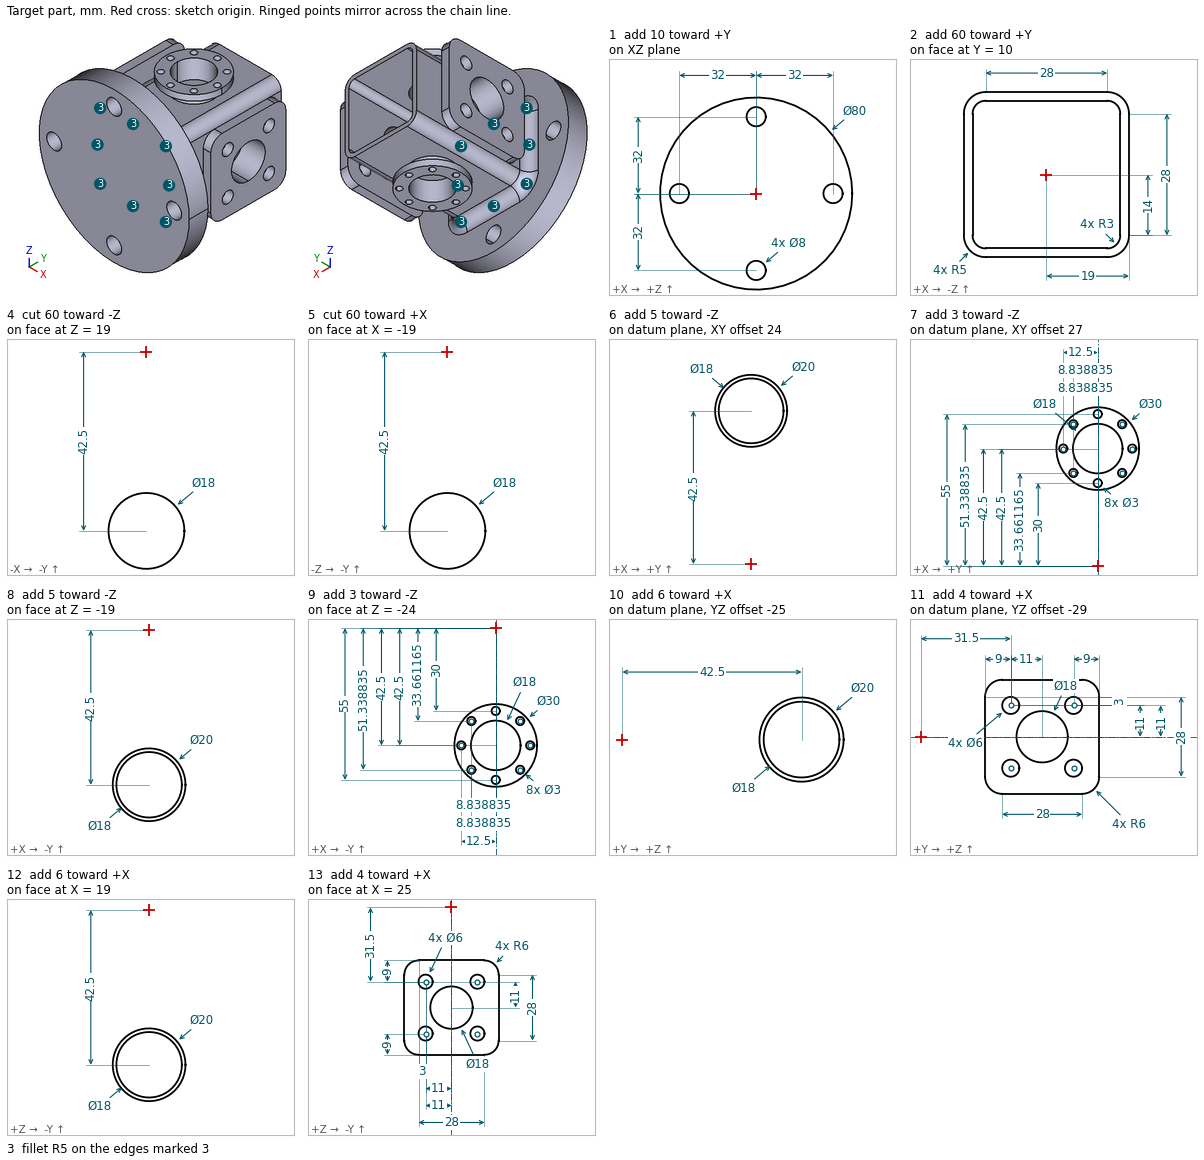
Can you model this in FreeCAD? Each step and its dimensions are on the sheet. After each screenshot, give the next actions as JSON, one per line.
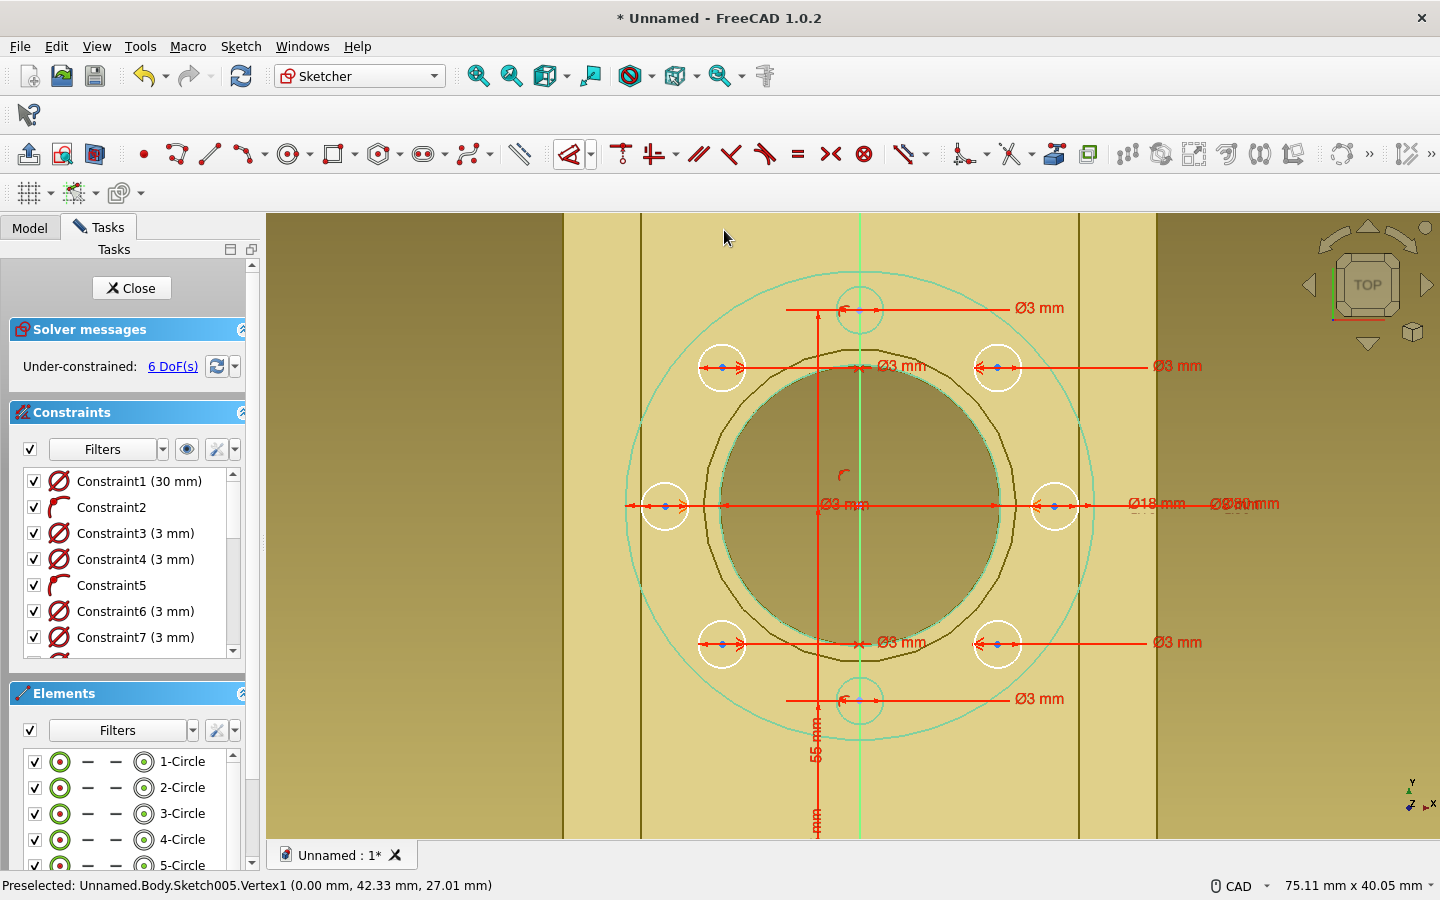
{"action": "left_click", "coordinate": [665, 506]}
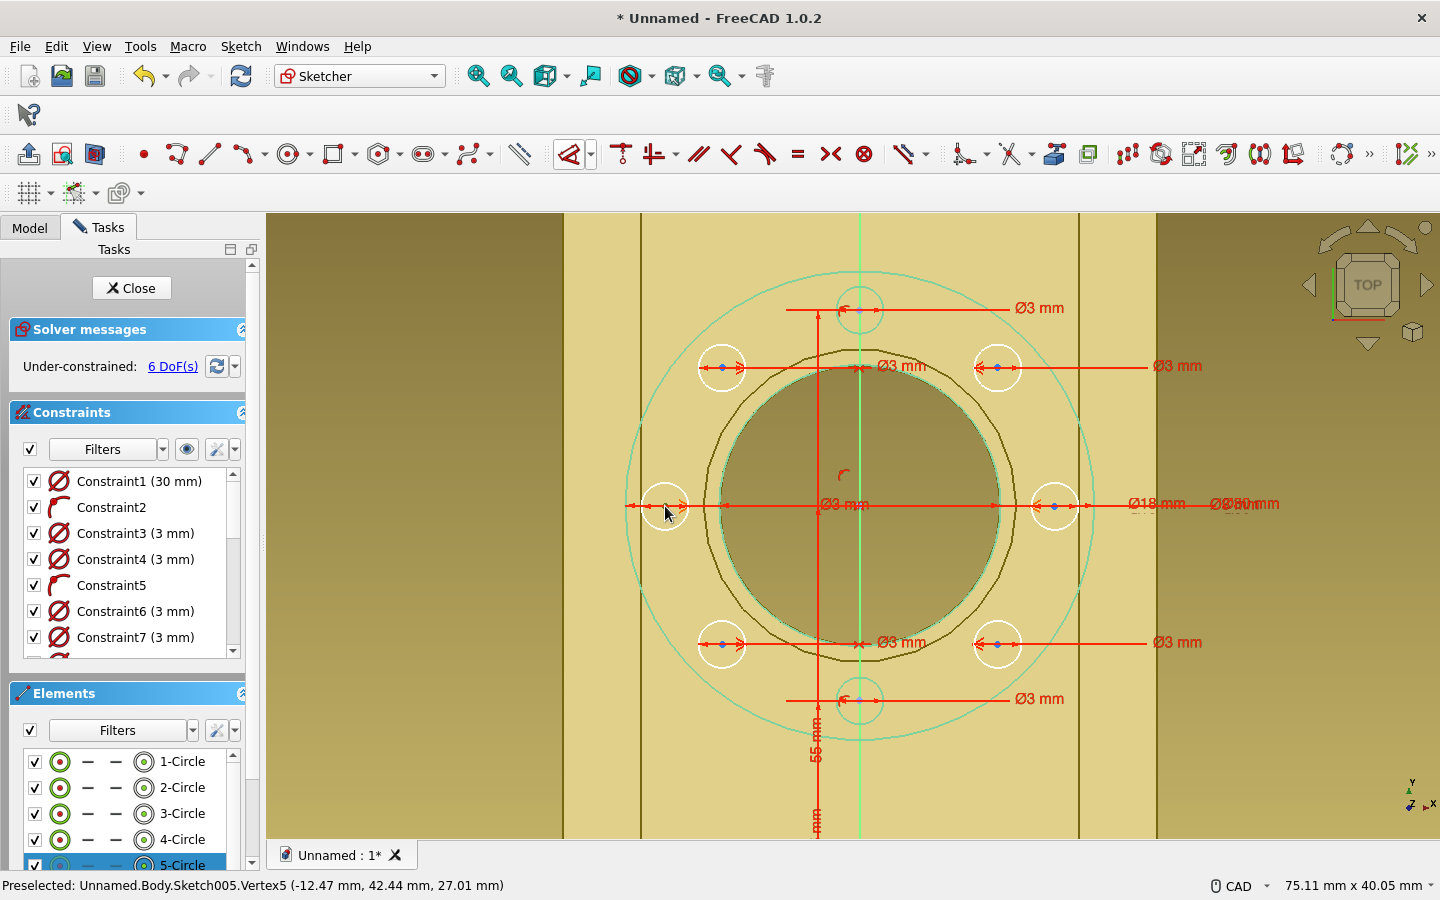
{"action": "key", "text": "l"}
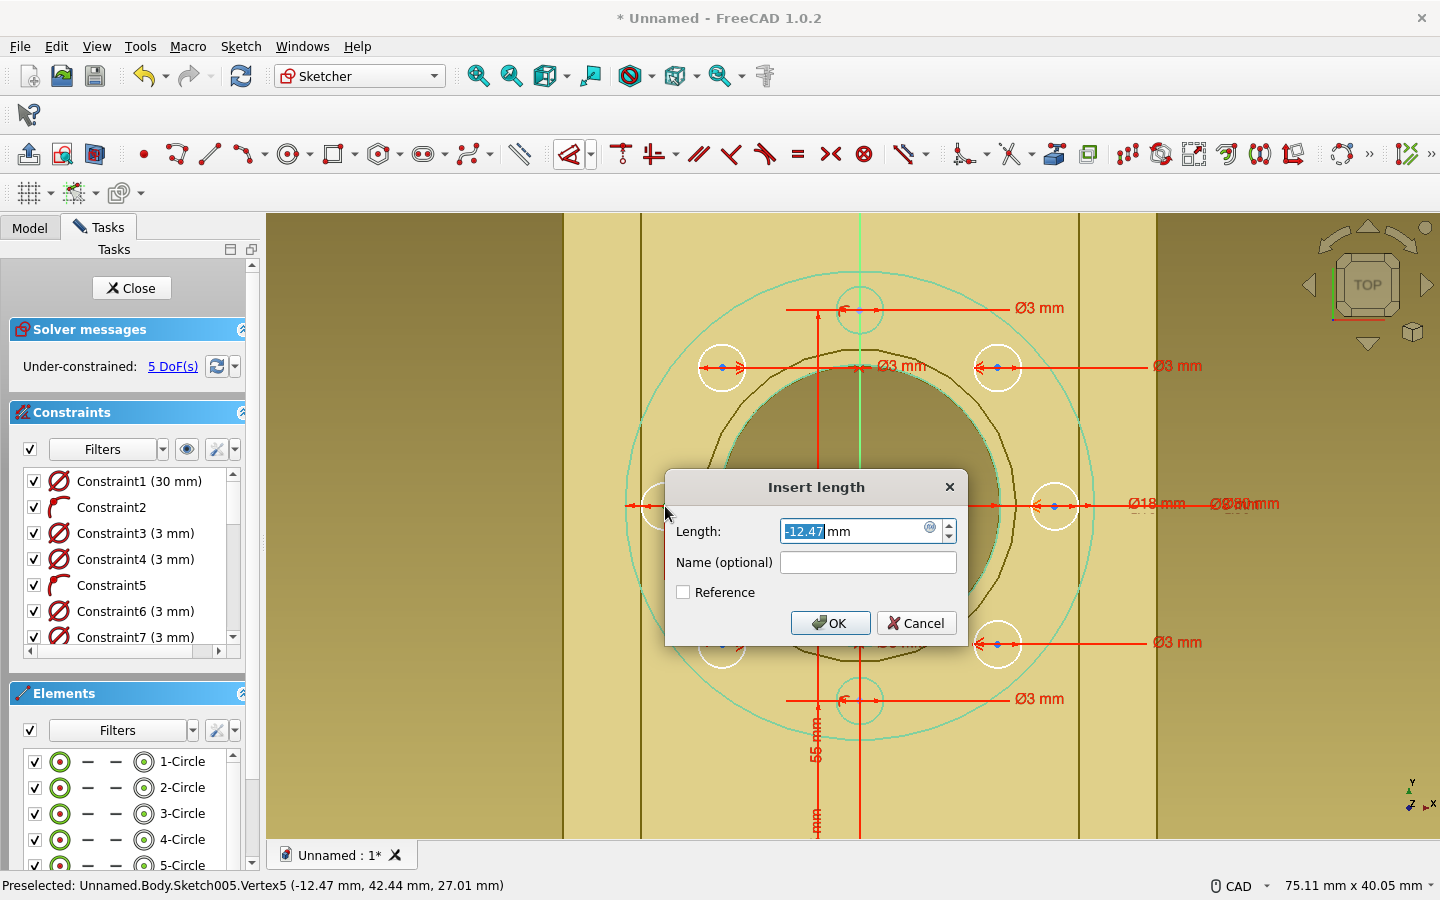
{"action": "type", "text": "-12.5"}
{"action": "key", "text": "Return"}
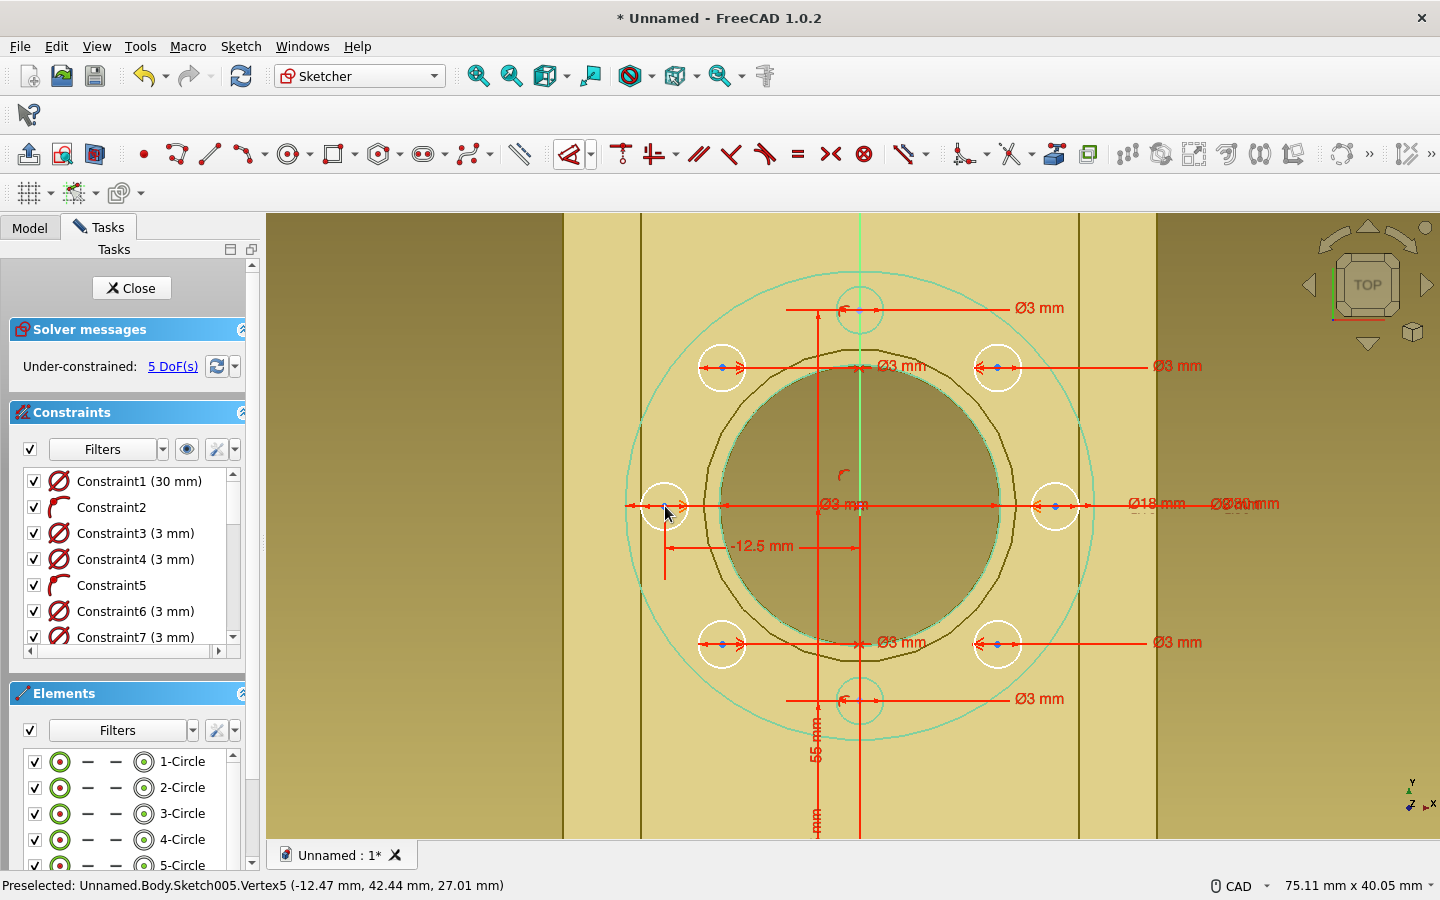
{"action": "left_click", "coordinate": [665, 506]}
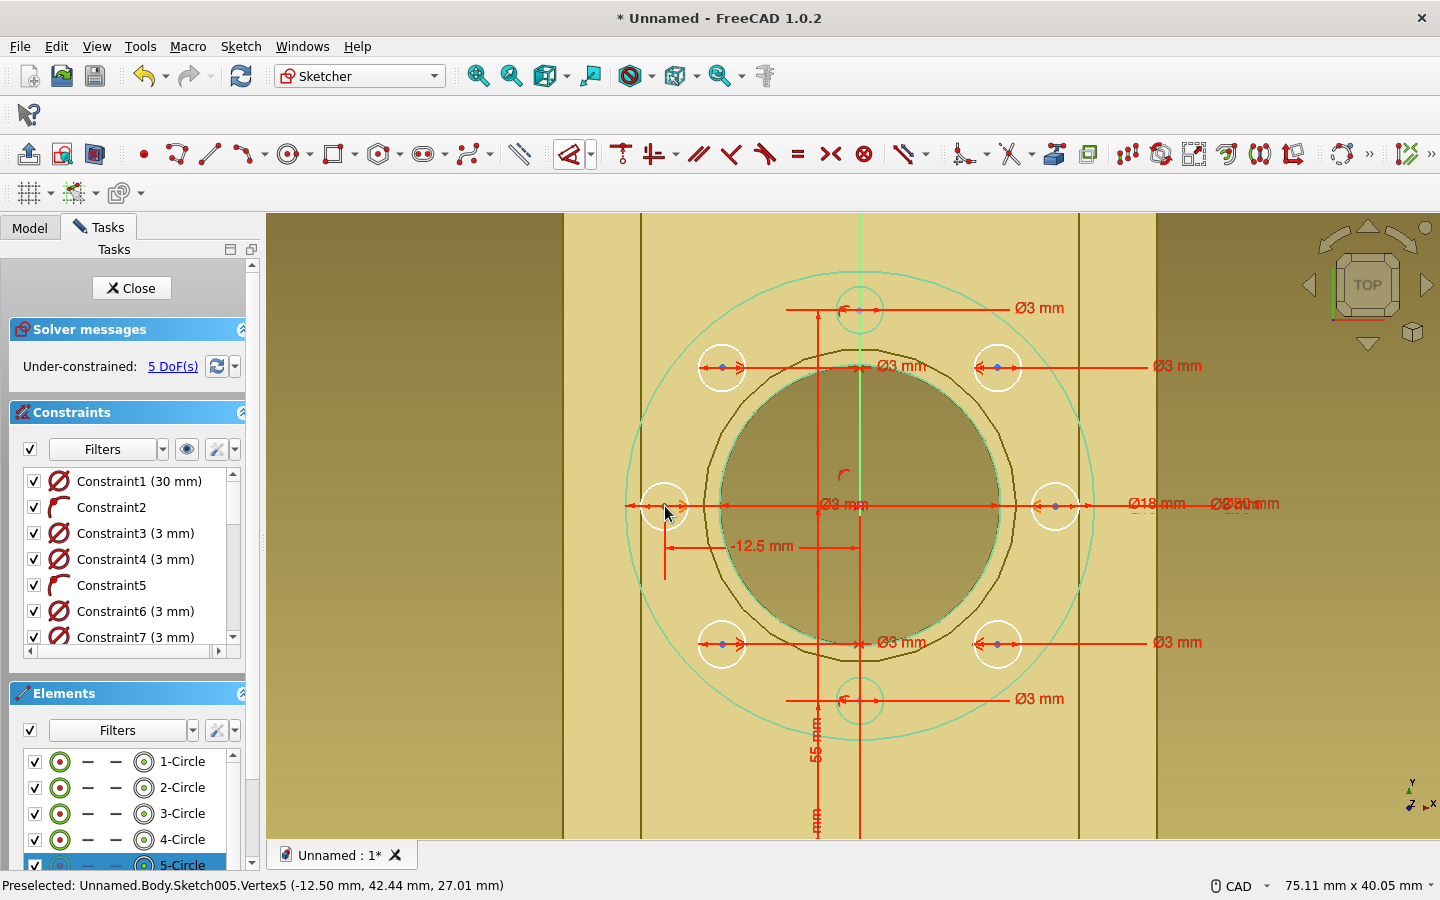
{"action": "left_click", "coordinate": [590, 154]}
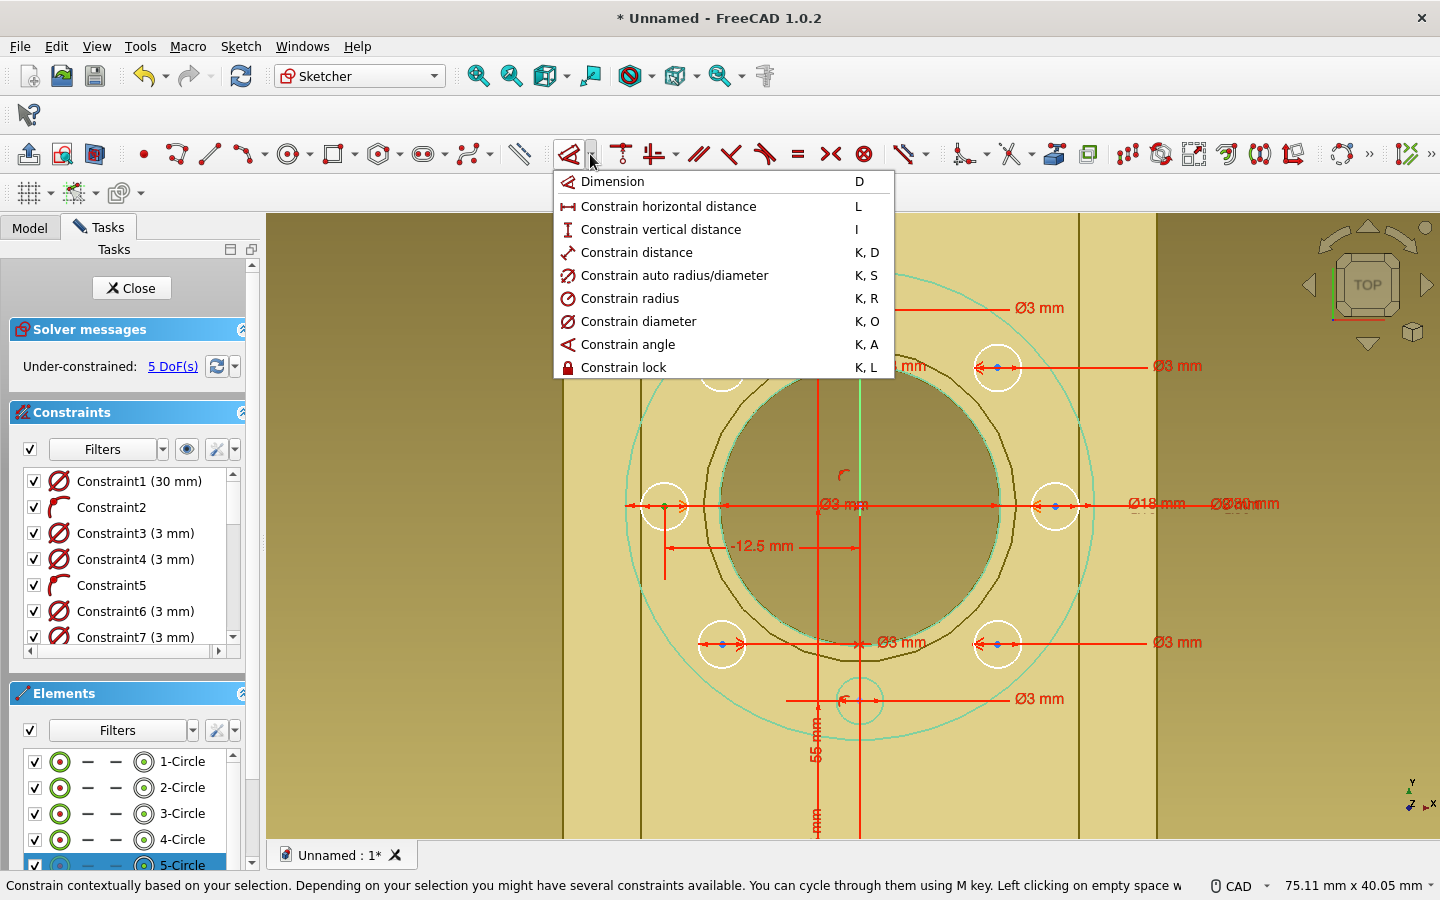
{"action": "left_click", "coordinate": [724, 230]}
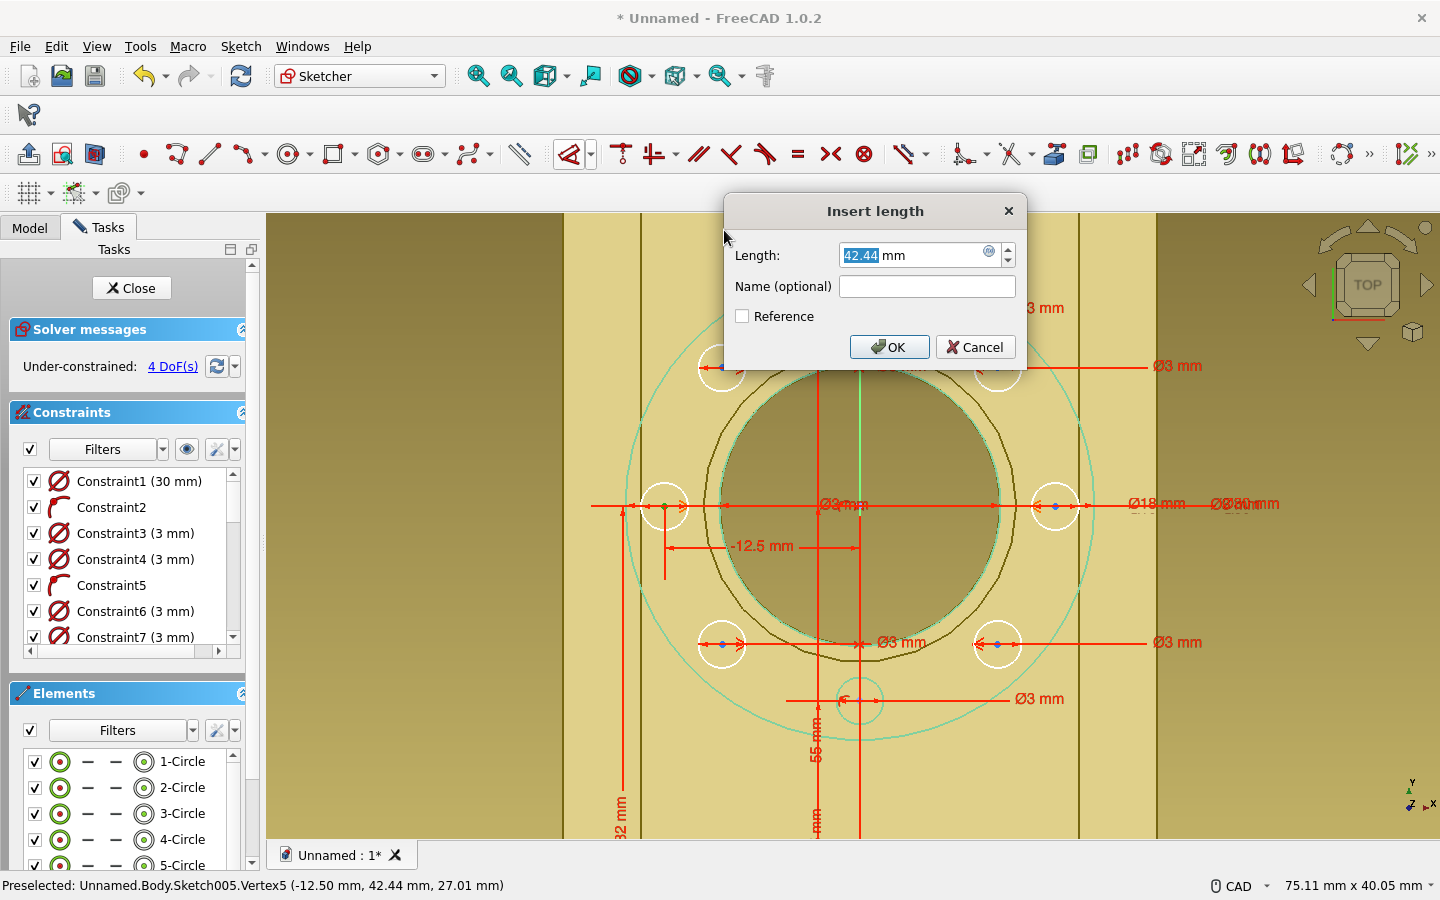
{"action": "type", "text": "42.5"}
{"action": "key", "text": "Return"}